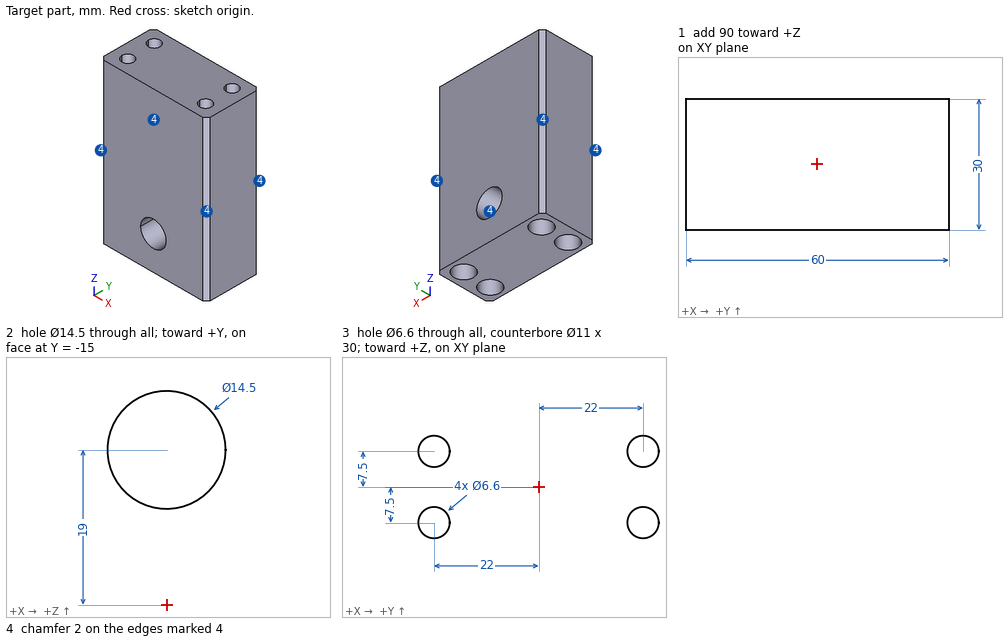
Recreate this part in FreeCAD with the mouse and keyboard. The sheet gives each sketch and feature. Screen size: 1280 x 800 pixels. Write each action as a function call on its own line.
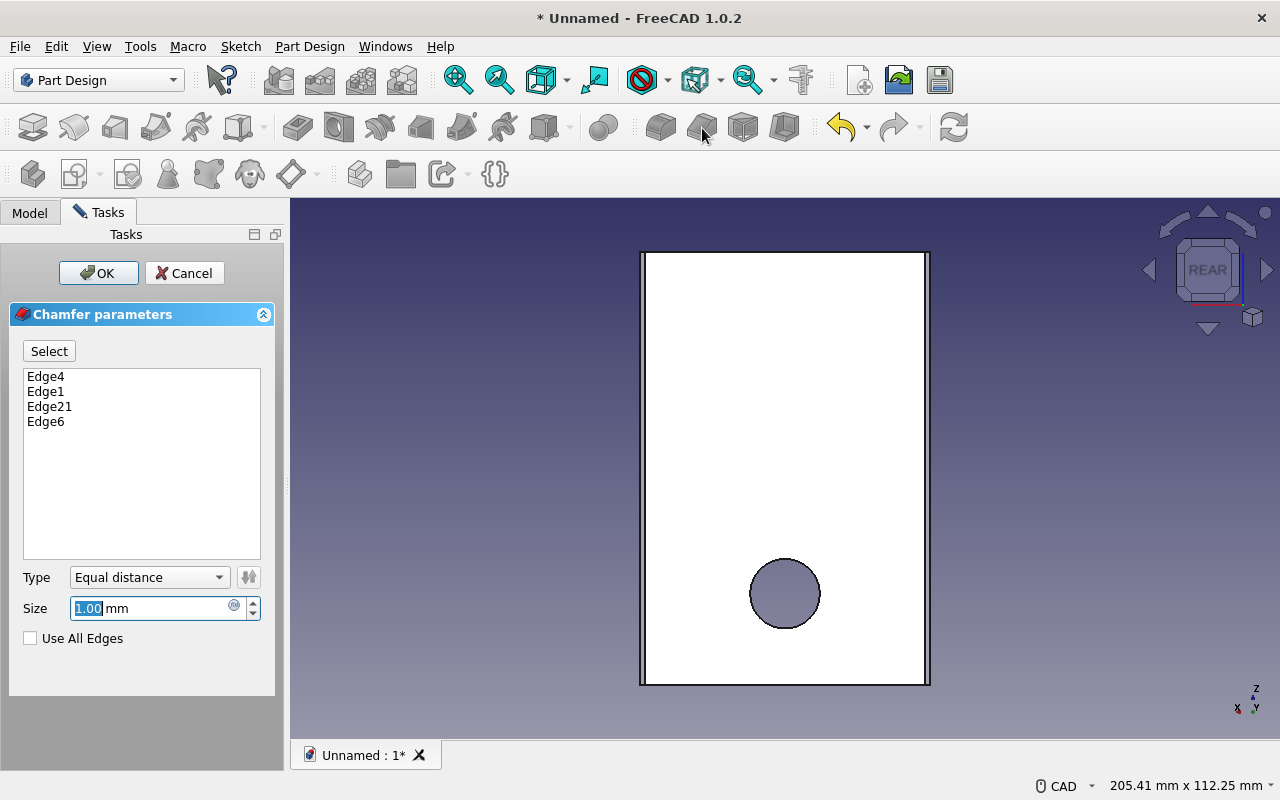
text(2)
key(Tab)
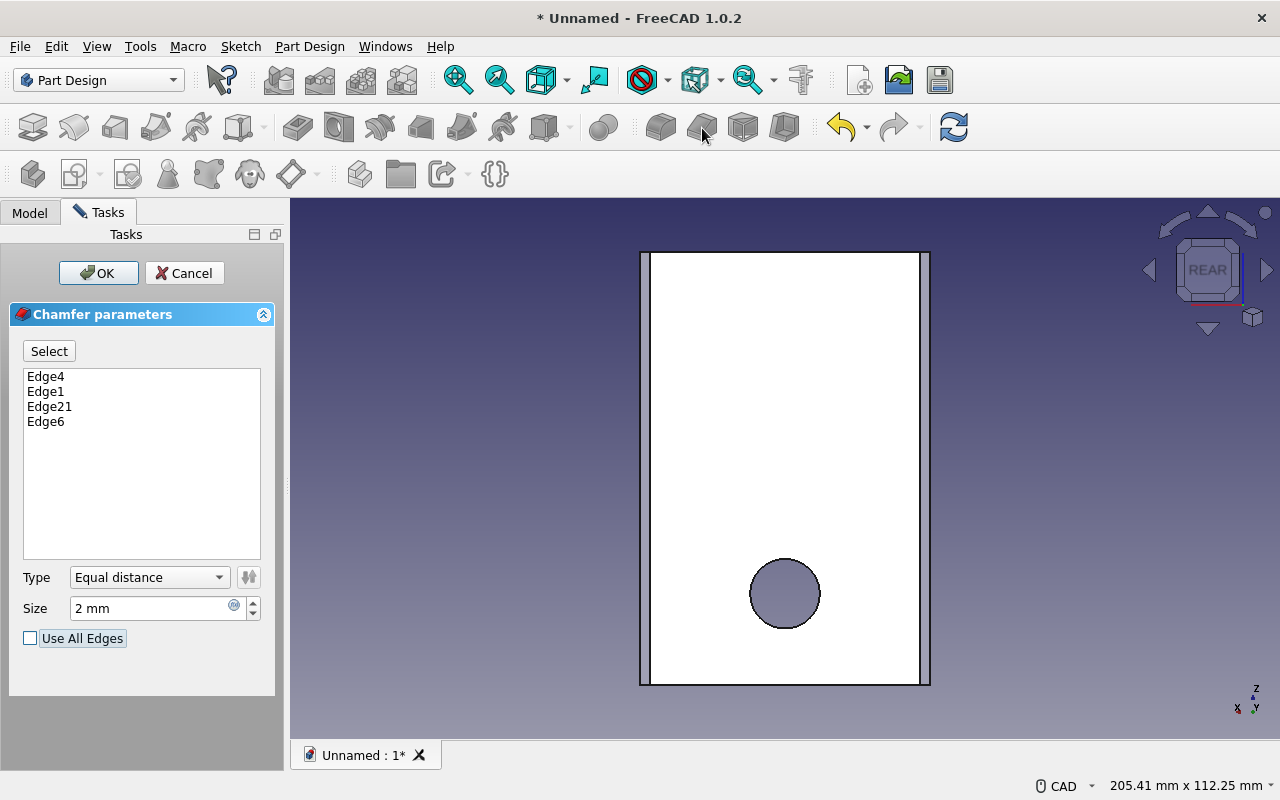
click(99, 273)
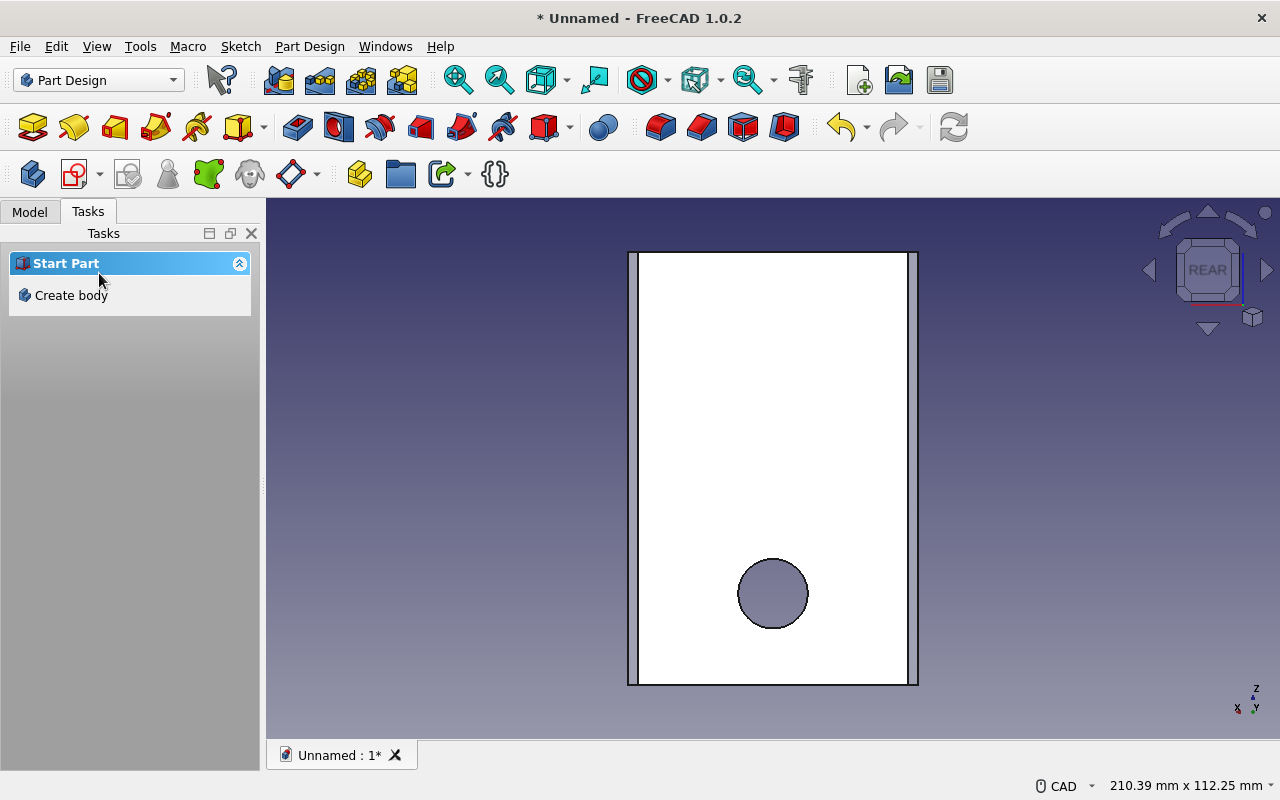
key(0)